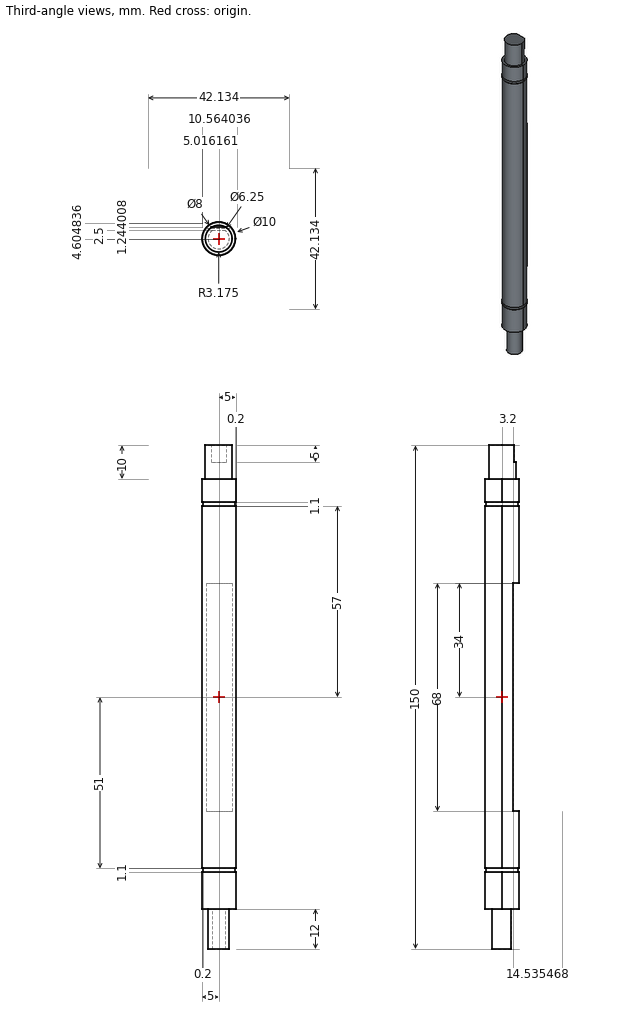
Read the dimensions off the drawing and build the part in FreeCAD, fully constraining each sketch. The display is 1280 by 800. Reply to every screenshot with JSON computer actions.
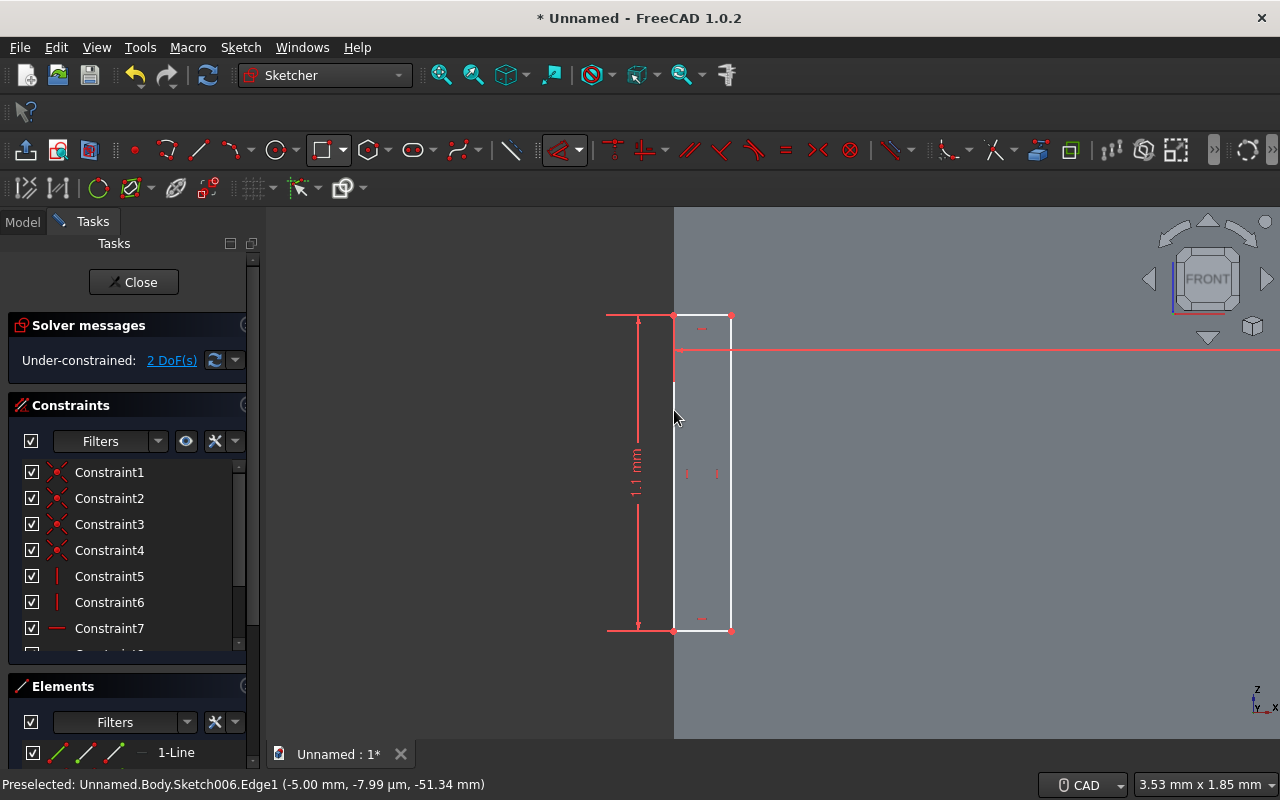
{"action": "left_click", "coordinate": [691, 631]}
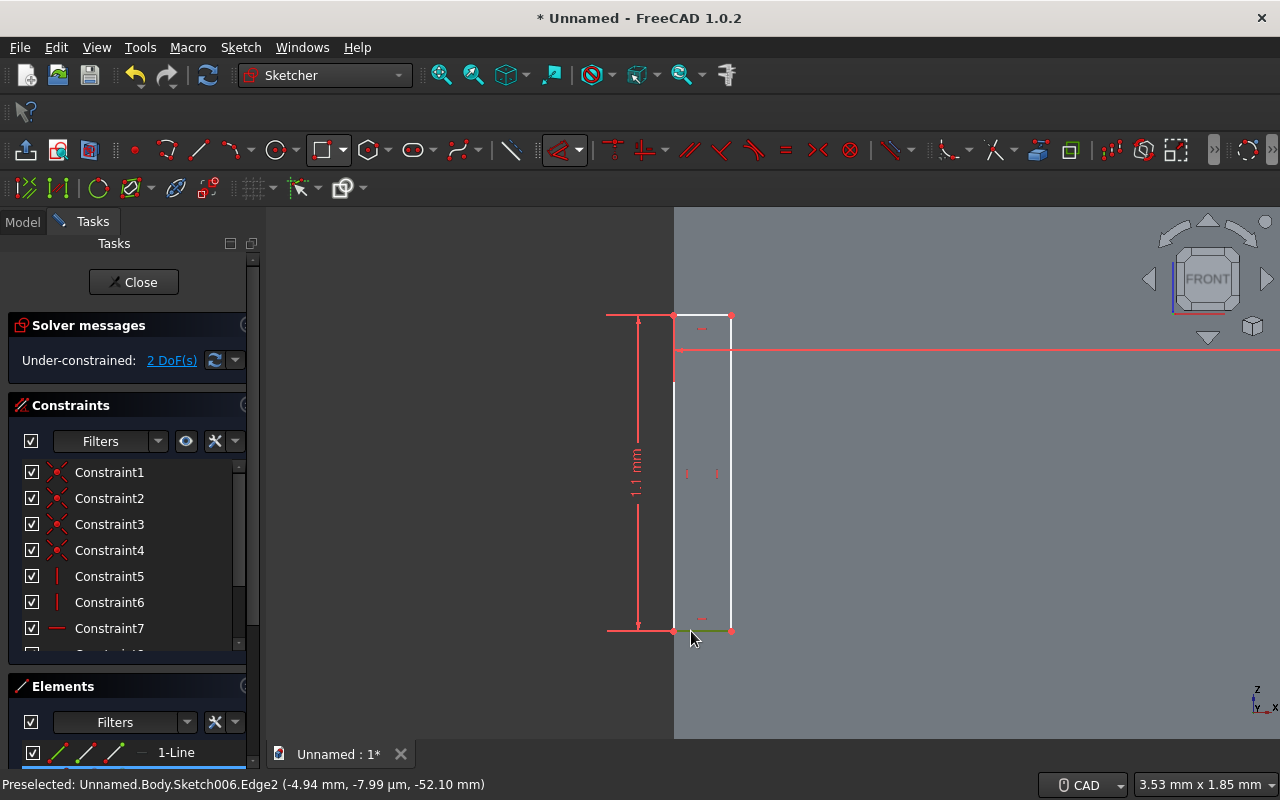
{"action": "left_click", "coordinate": [582, 150]}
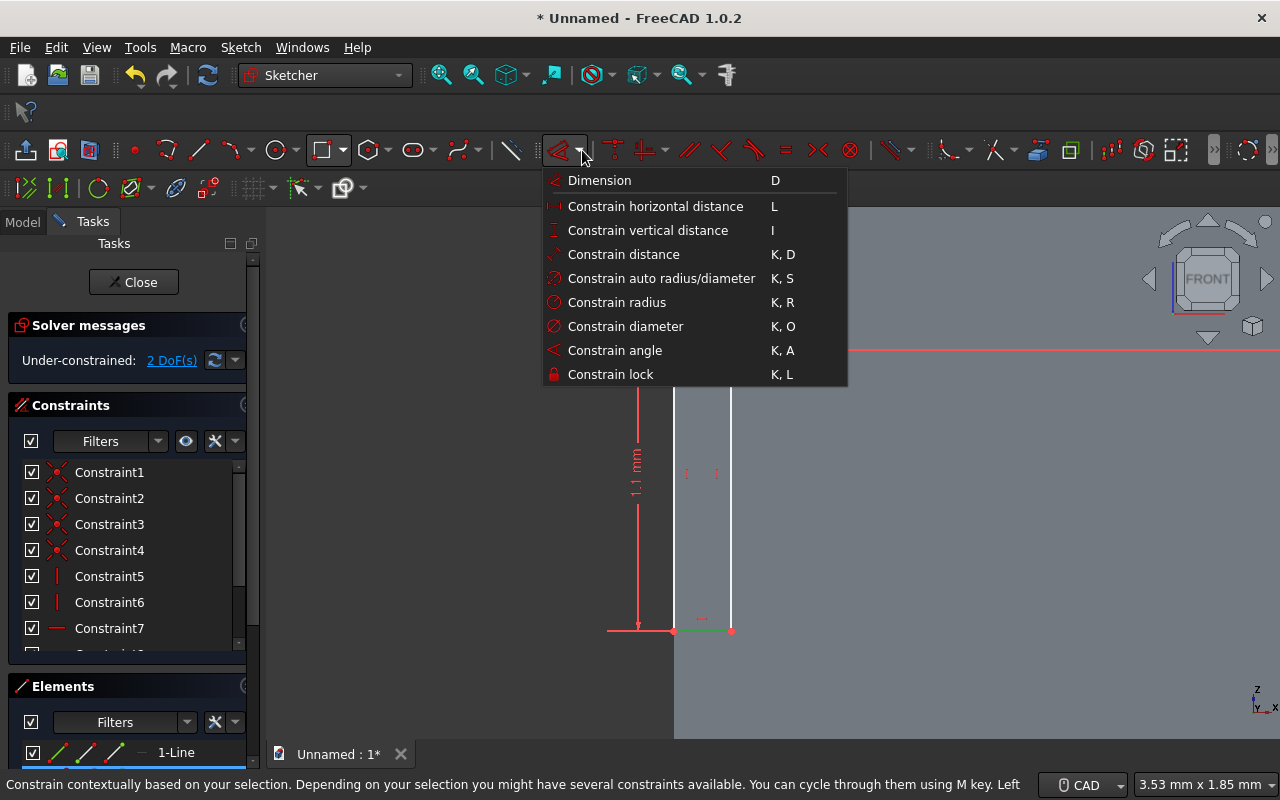
{"action": "left_click", "coordinate": [695, 206]}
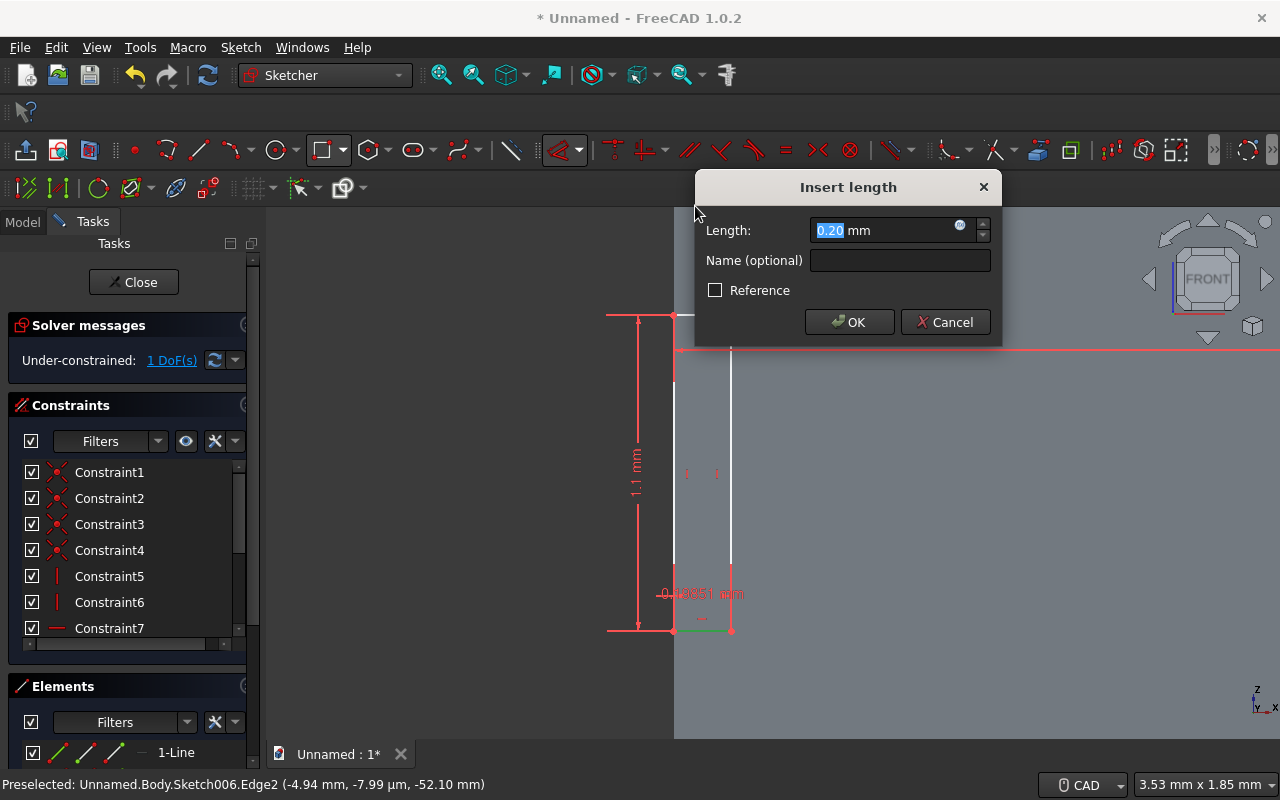
{"action": "type", "text": "0.2"}
{"action": "key", "text": "Return"}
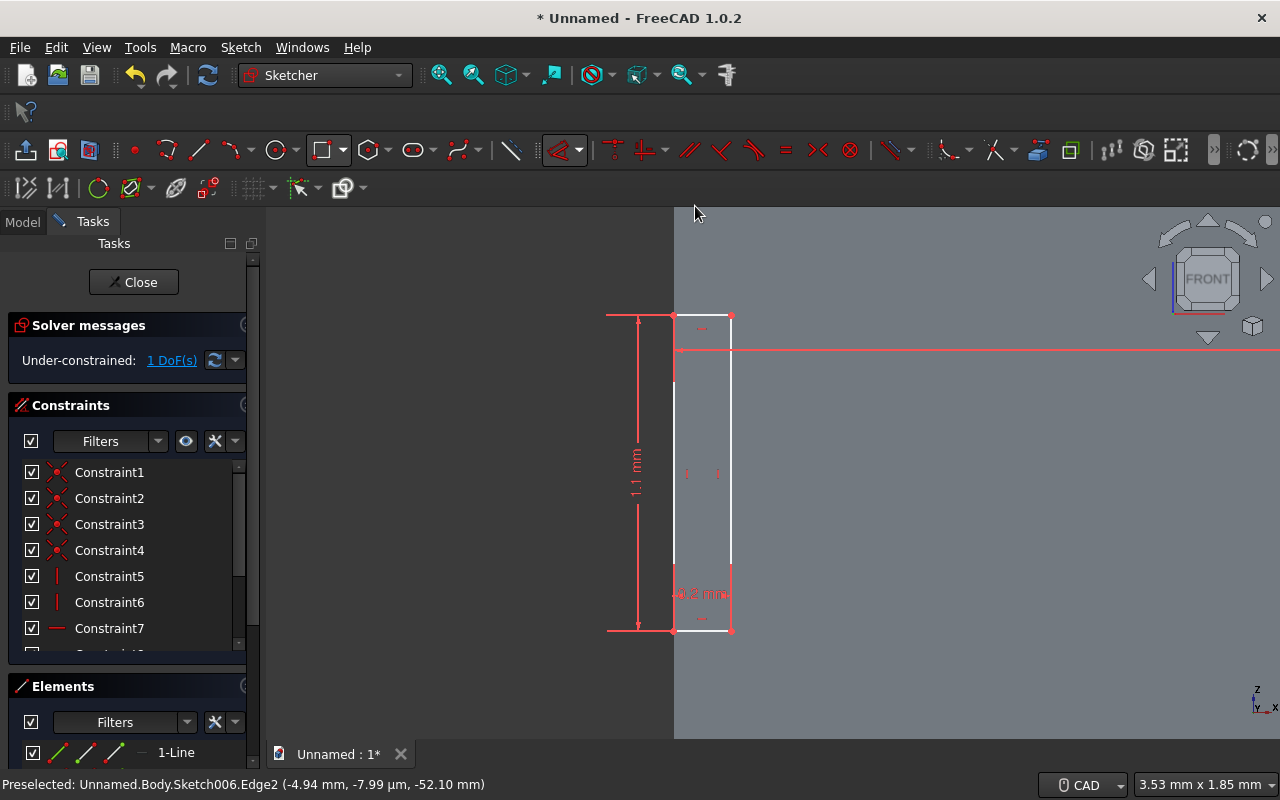
{"action": "left_click", "coordinate": [674, 315]}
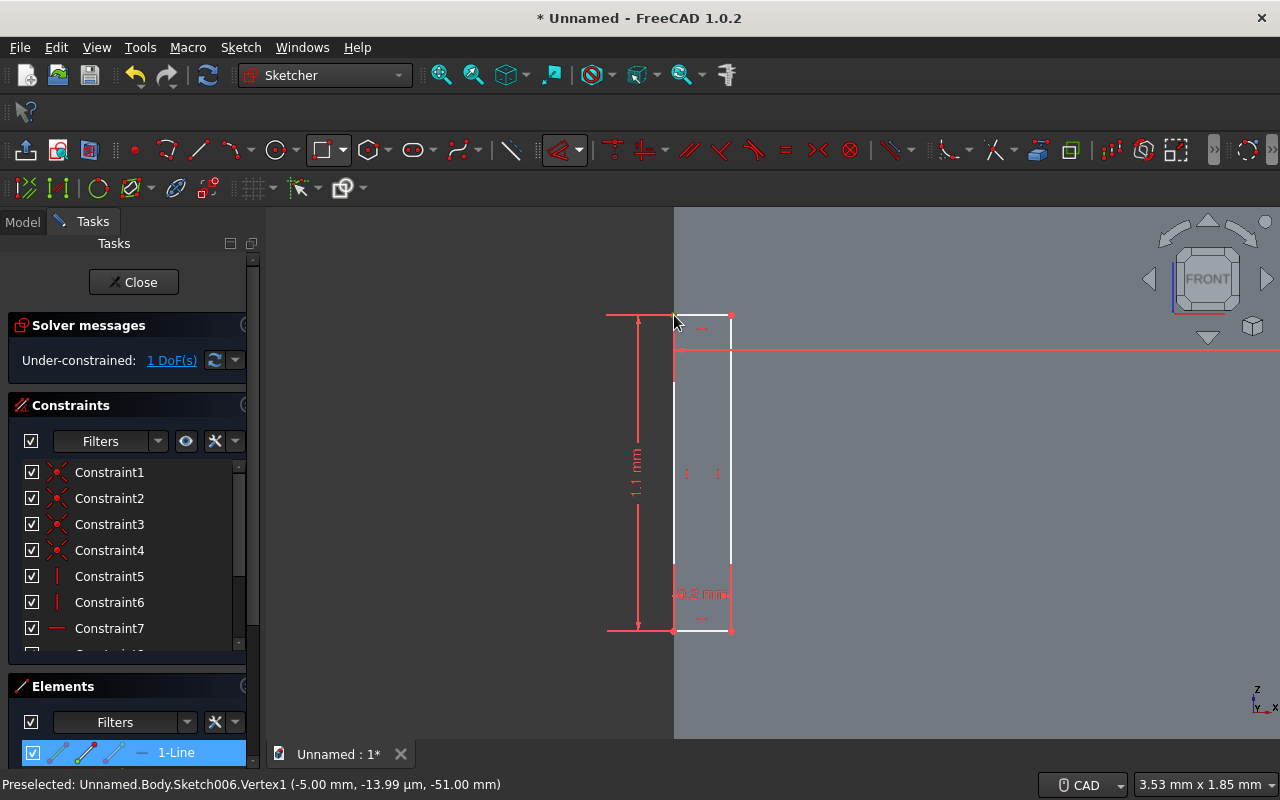
{"action": "left_click", "coordinate": [582, 150]}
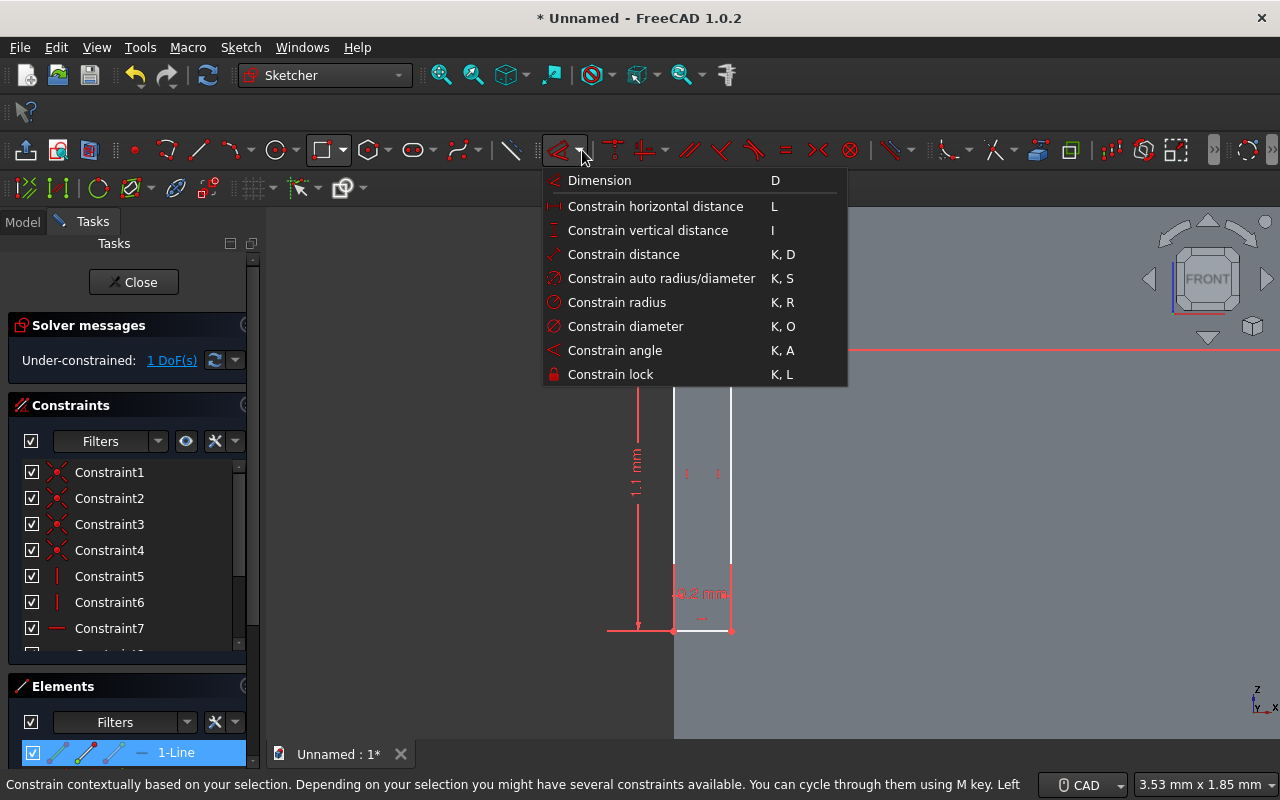
{"action": "left_click", "coordinate": [695, 230]}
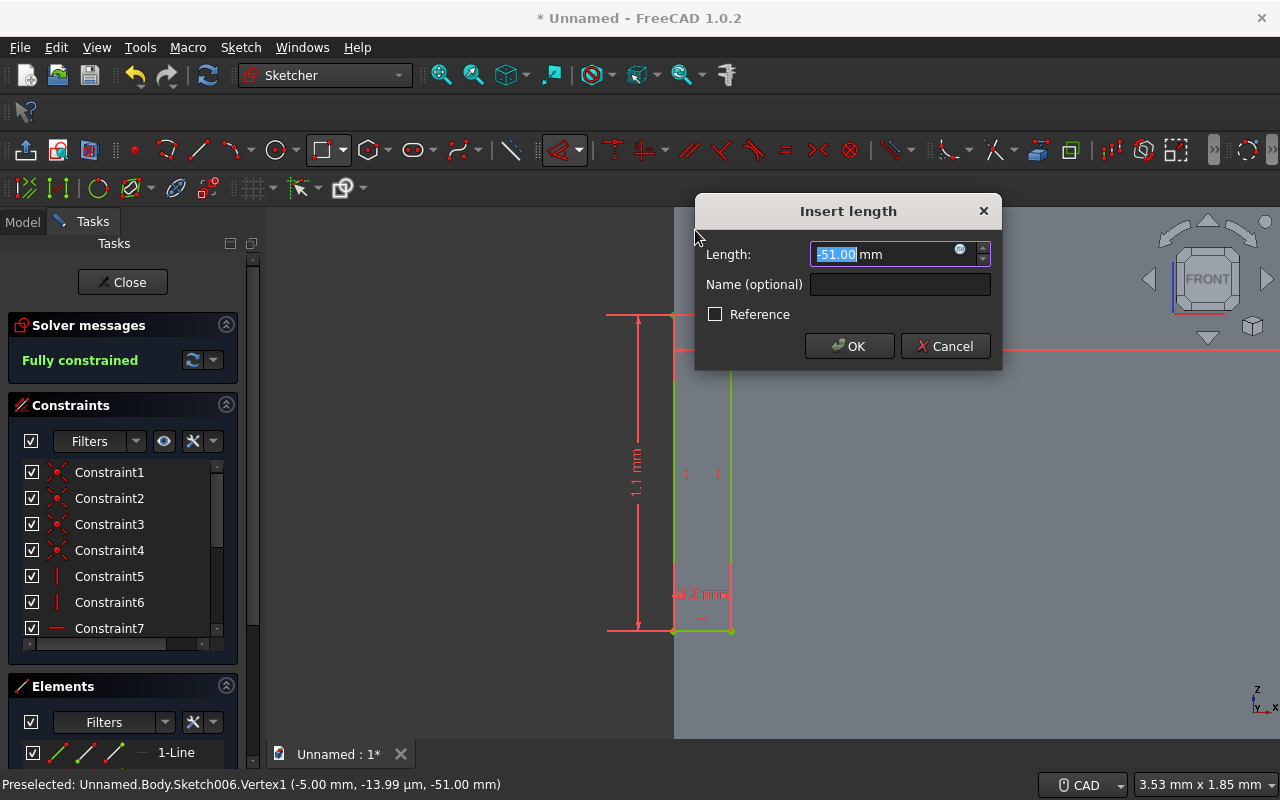
{"action": "type", "text": "-51"}
{"action": "key", "text": "Return"}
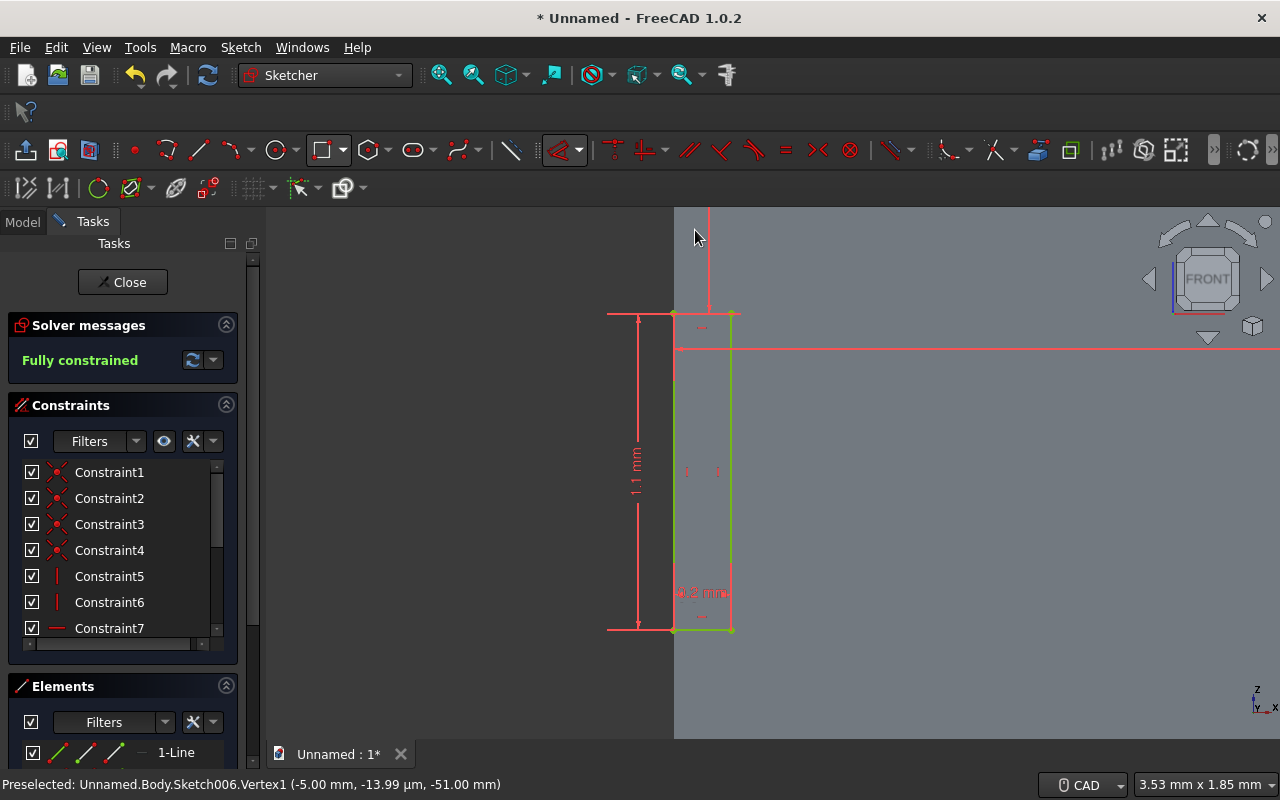
{"action": "left_click", "coordinate": [123, 282]}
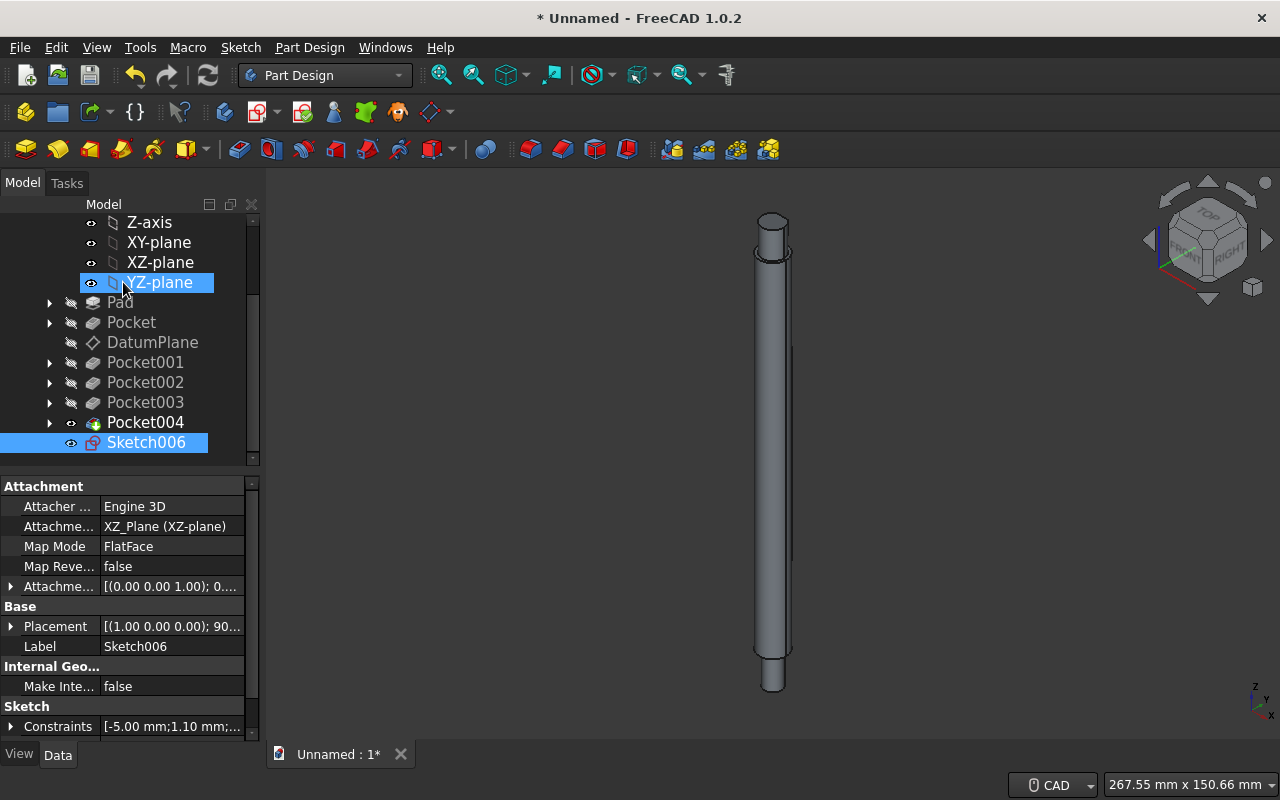
{"action": "left_click", "coordinate": [304, 150]}